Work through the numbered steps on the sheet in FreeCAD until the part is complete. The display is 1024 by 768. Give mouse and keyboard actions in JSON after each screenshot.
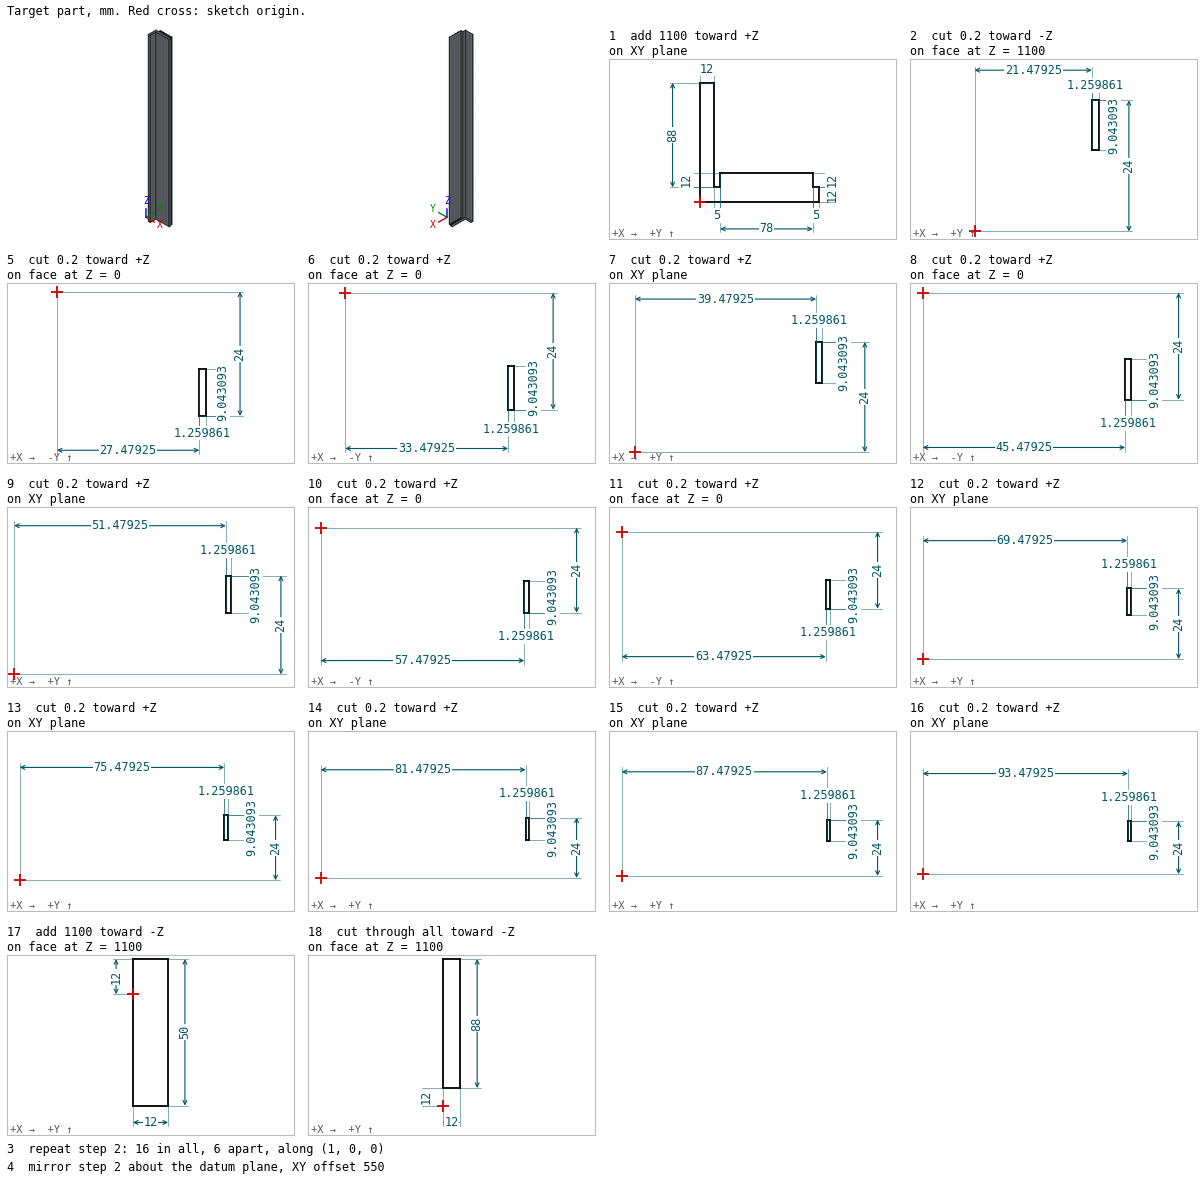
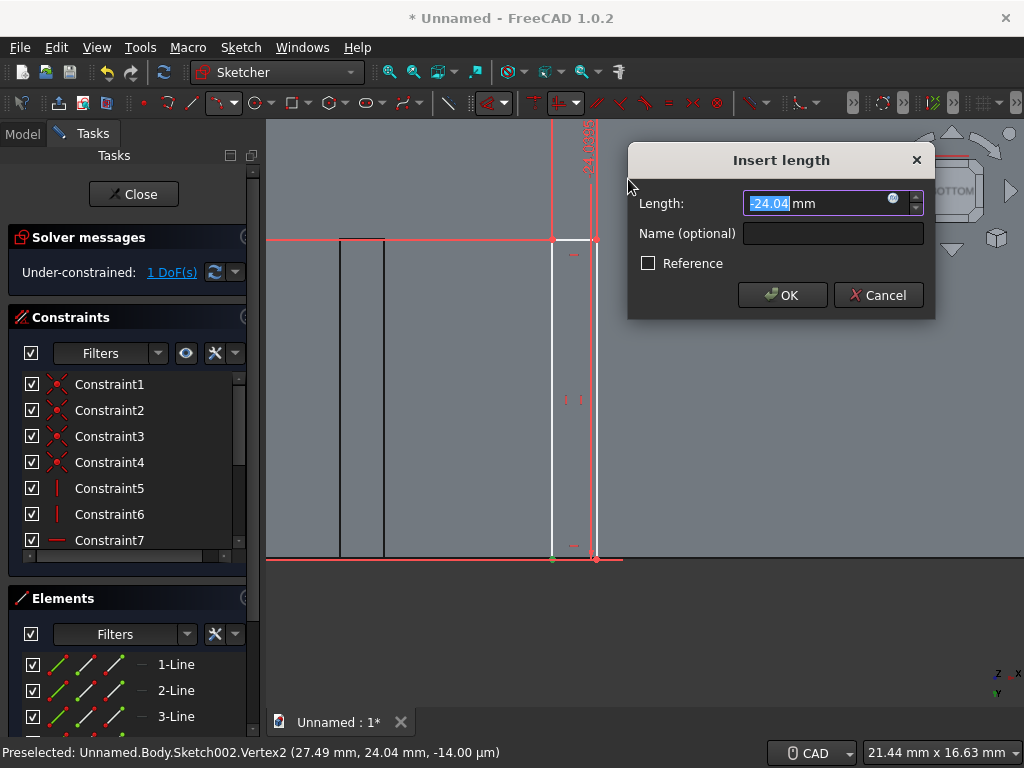
{"action": "type", "text": "-24"}
{"action": "key", "text": "Return"}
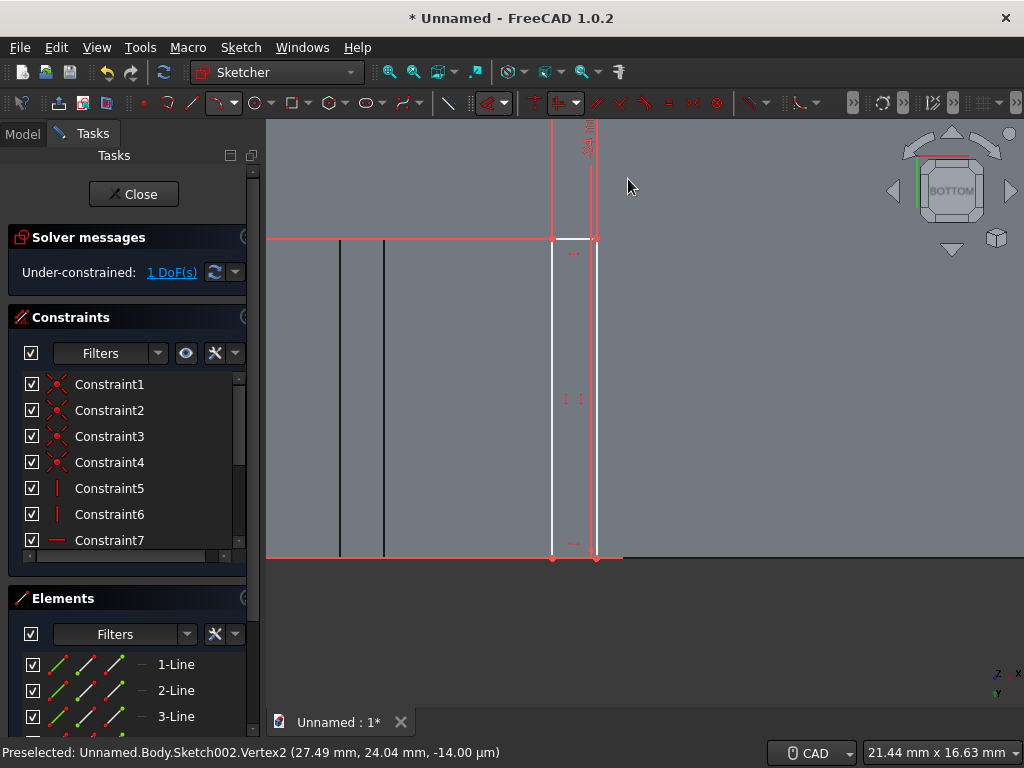
{"action": "left_click", "coordinate": [552, 239]}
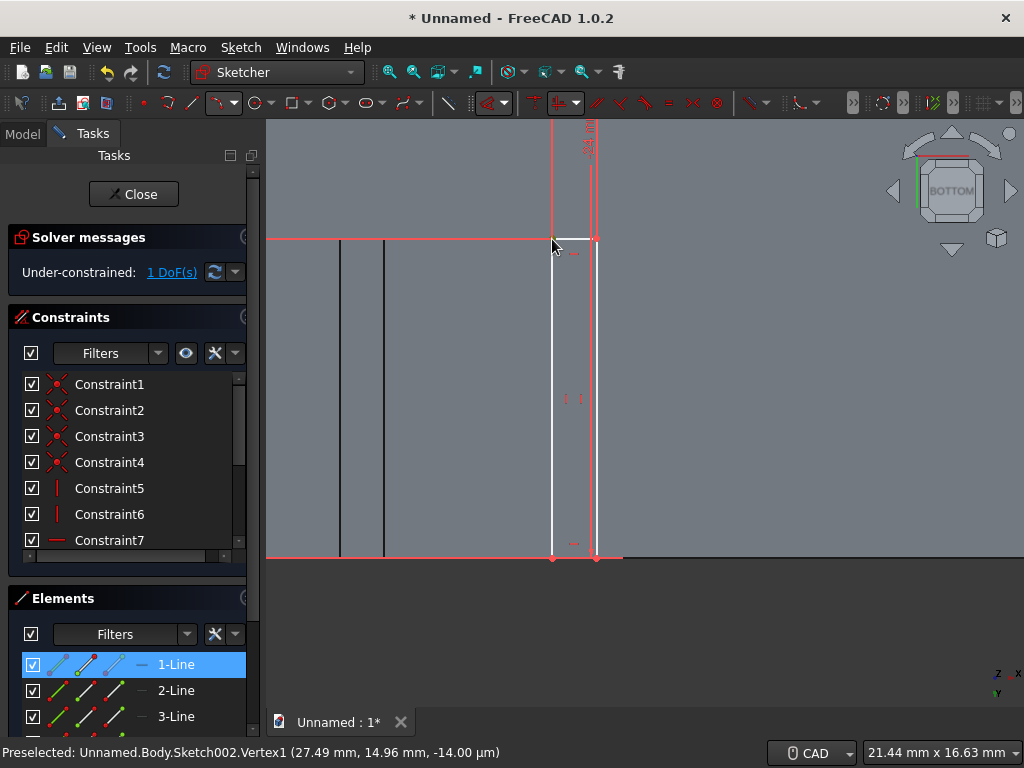
{"action": "key", "text": "l"}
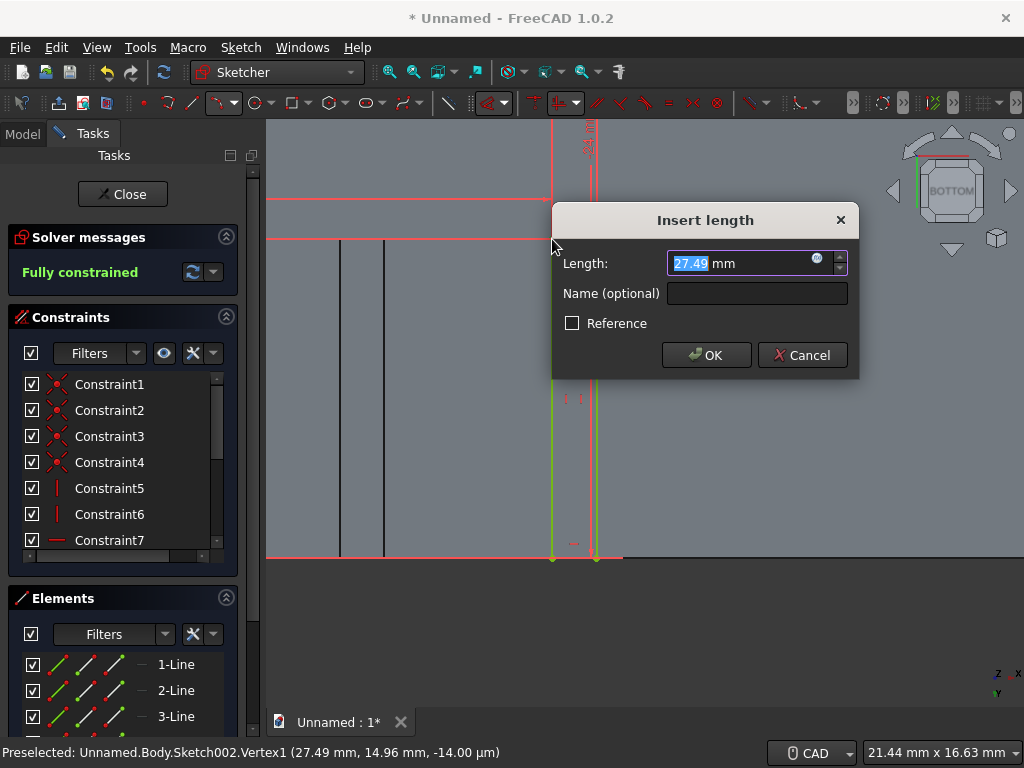
{"action": "type", "text": "27.47925"}
{"action": "key", "text": "Return"}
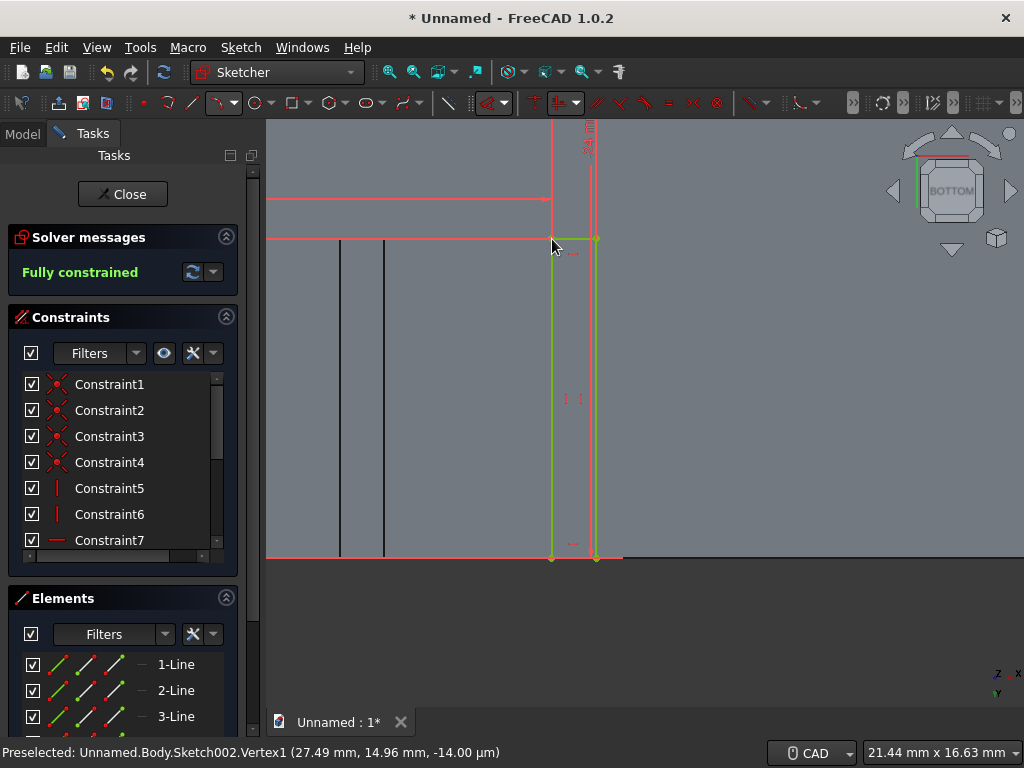
{"action": "left_click", "coordinate": [123, 194]}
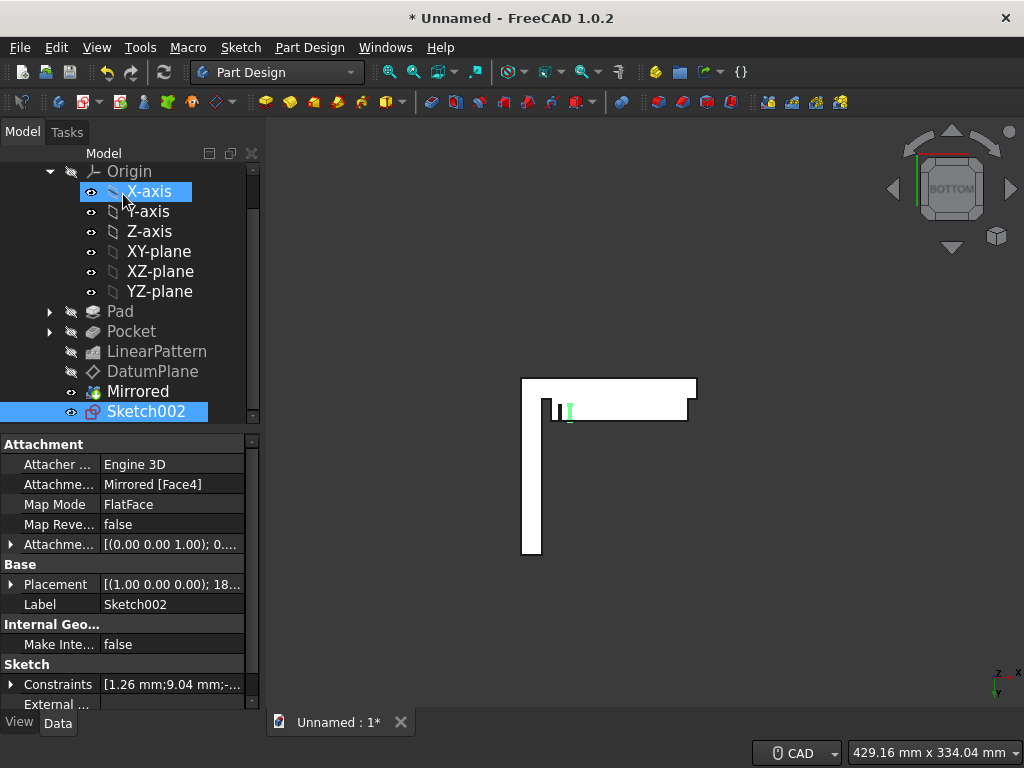
{"action": "left_click", "coordinate": [432, 102]}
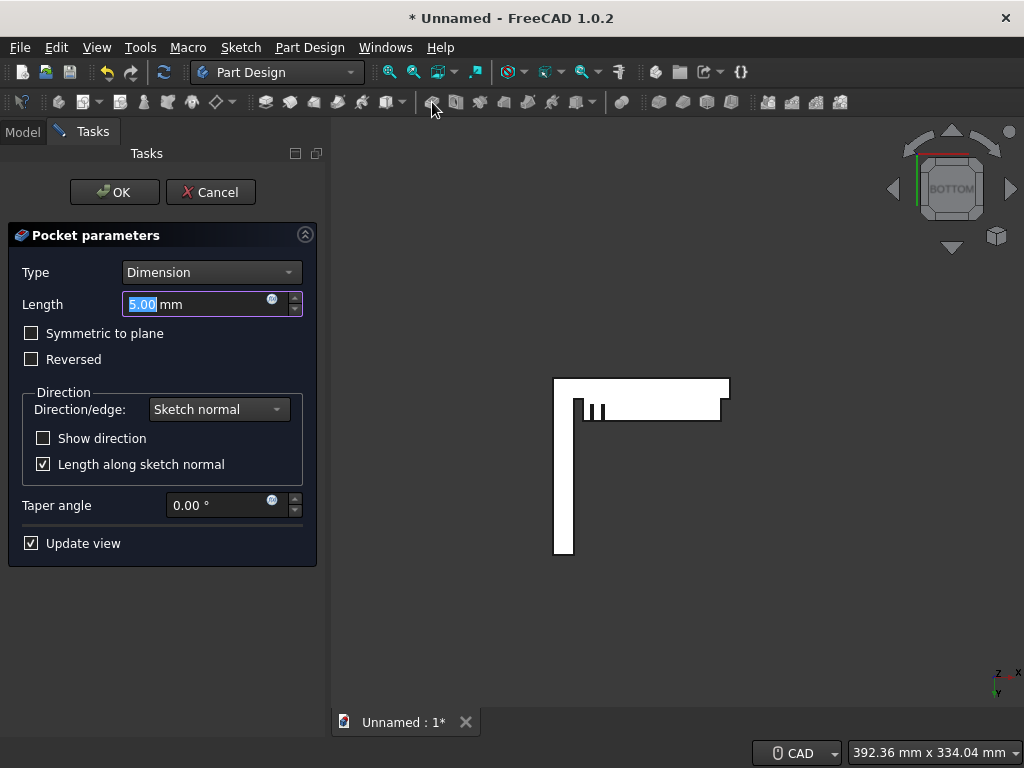
{"action": "type", "text": "0.2"}
{"action": "key", "text": "Tab"}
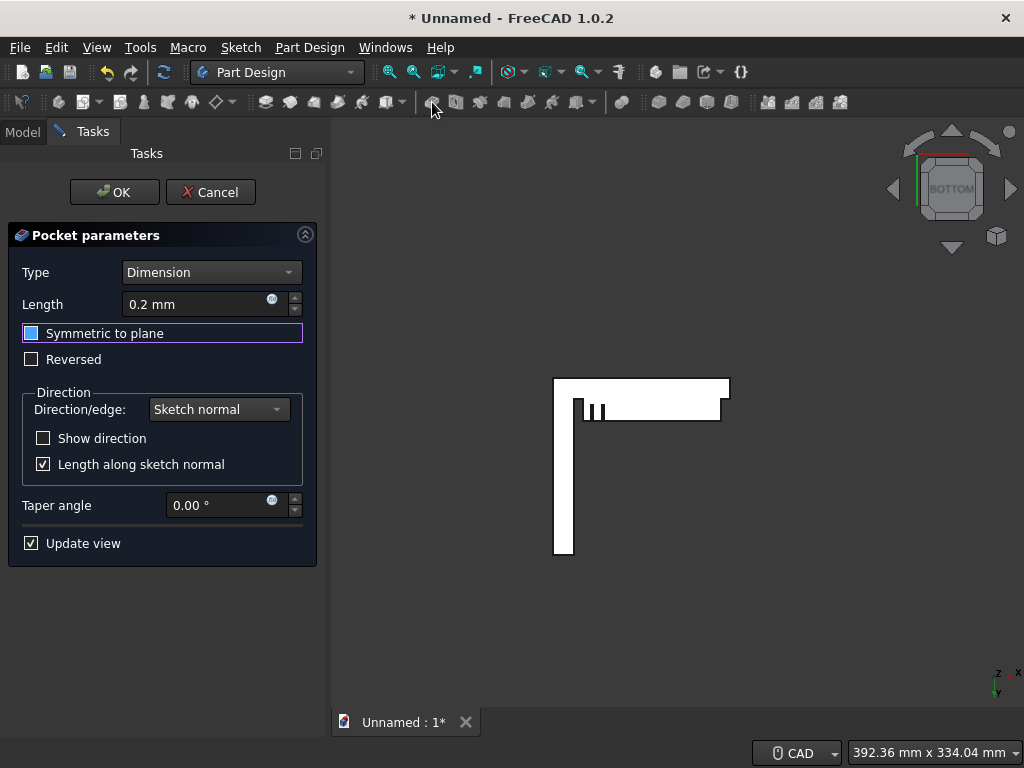
{"action": "left_click", "coordinate": [115, 192]}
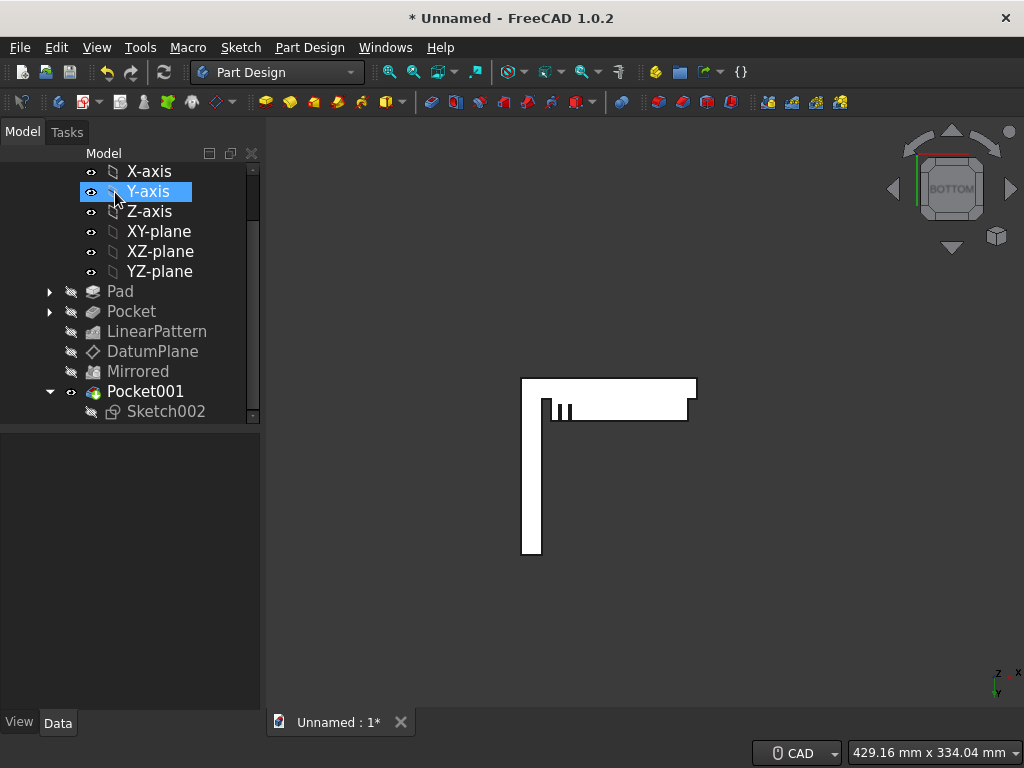
{"action": "left_click", "coordinate": [390, 72]}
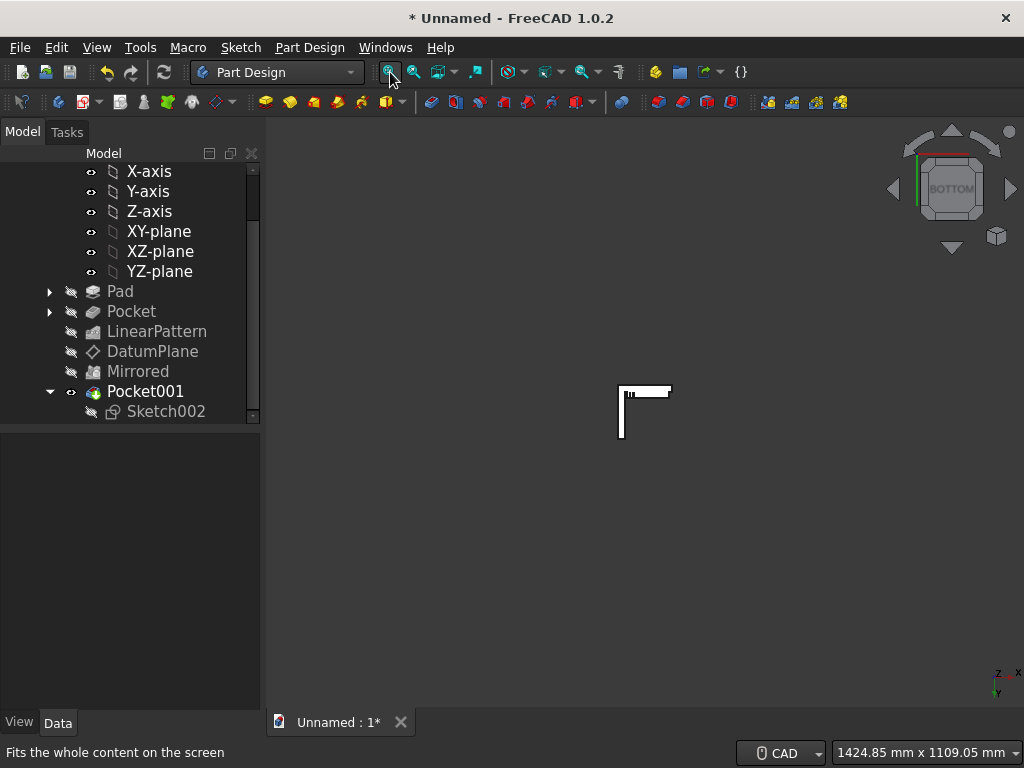
{"action": "left_click", "coordinate": [660, 388]}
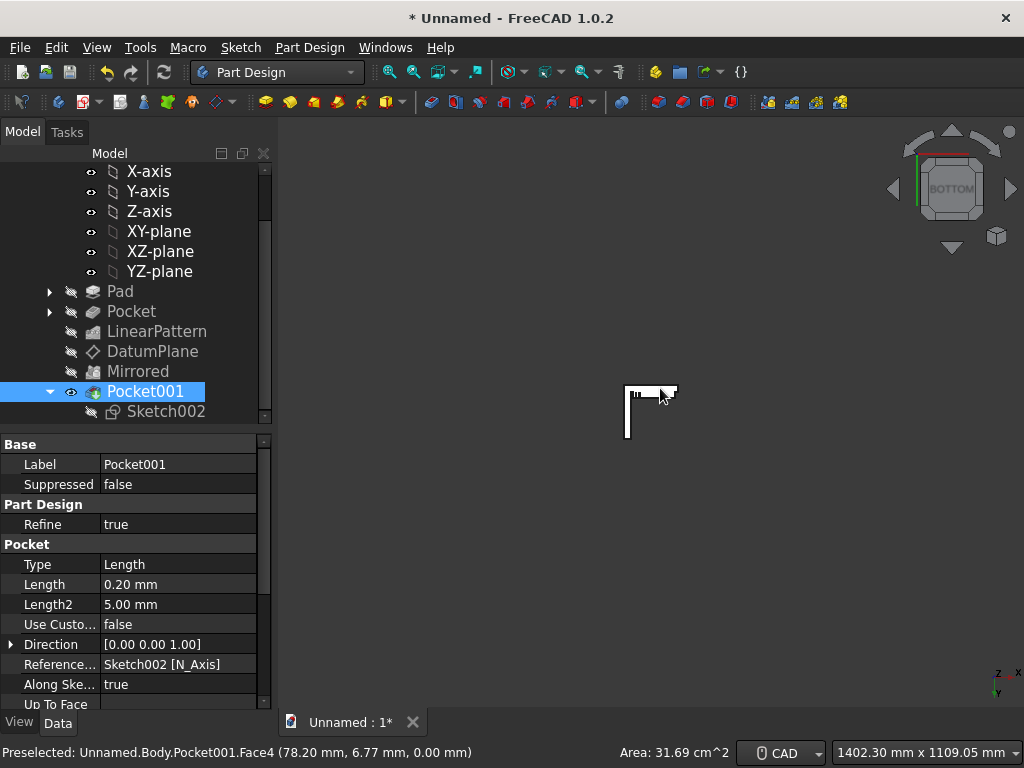
{"action": "left_click", "coordinate": [84, 102]}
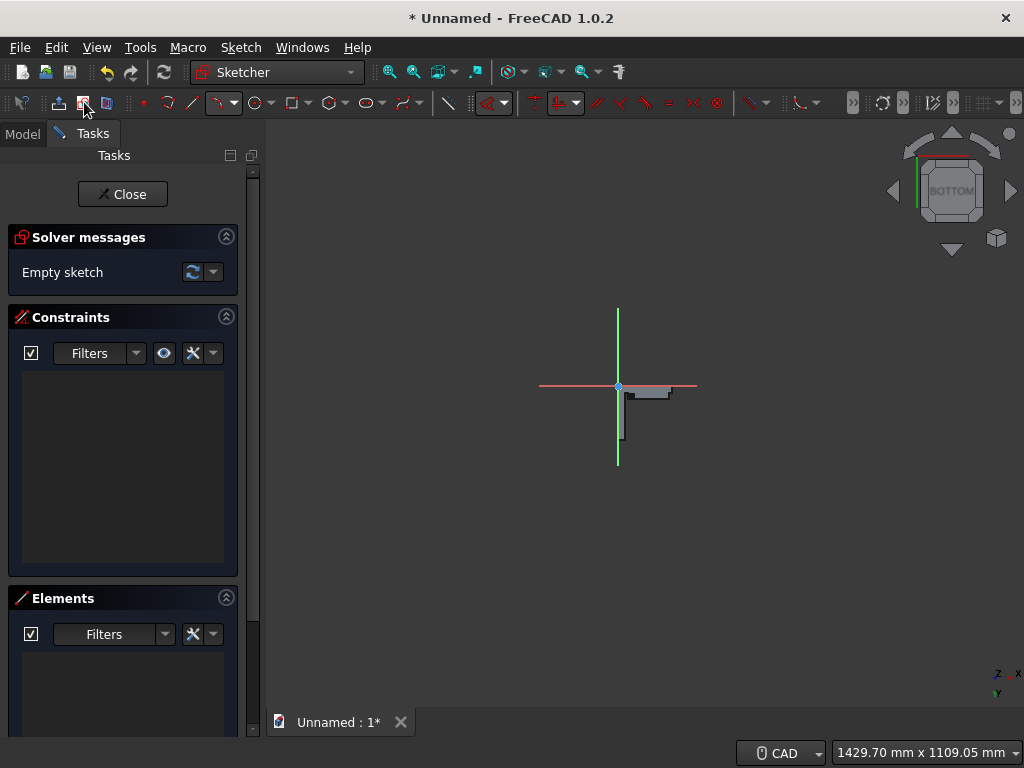
{"action": "scroll", "coordinate": [640, 396], "scroll_direction": "up", "scroll_amount": 15}